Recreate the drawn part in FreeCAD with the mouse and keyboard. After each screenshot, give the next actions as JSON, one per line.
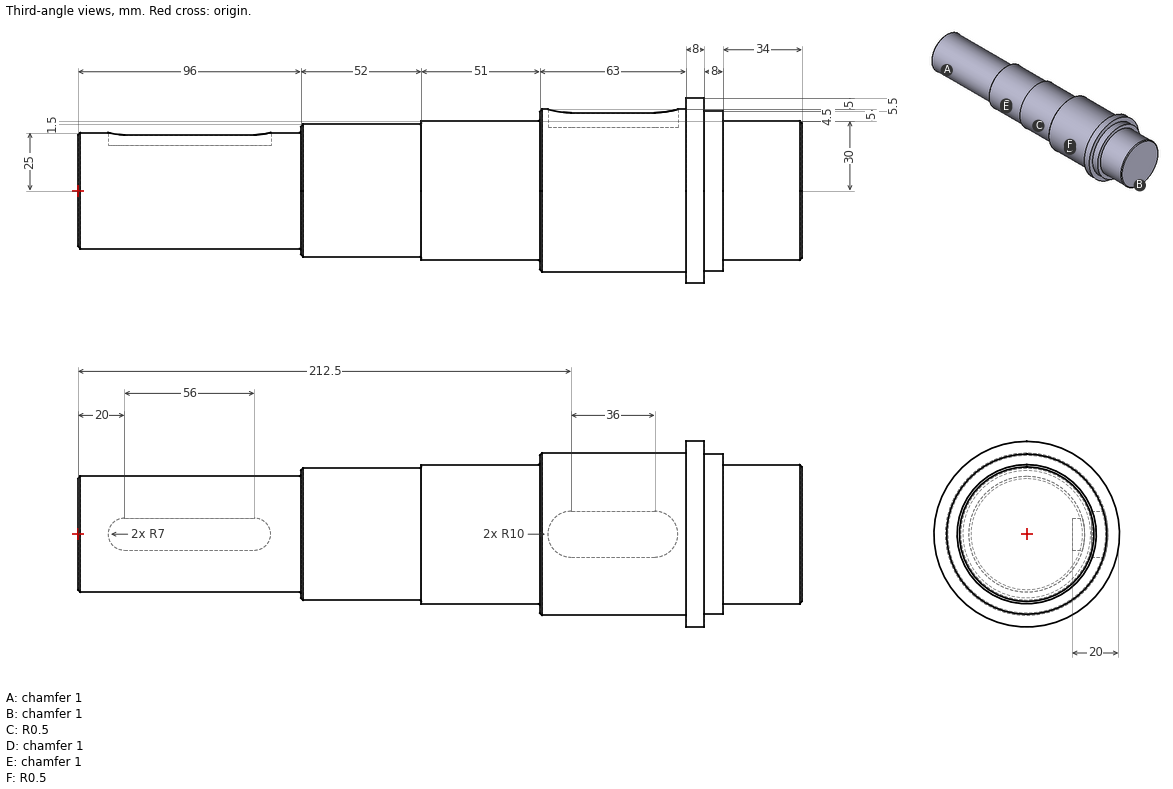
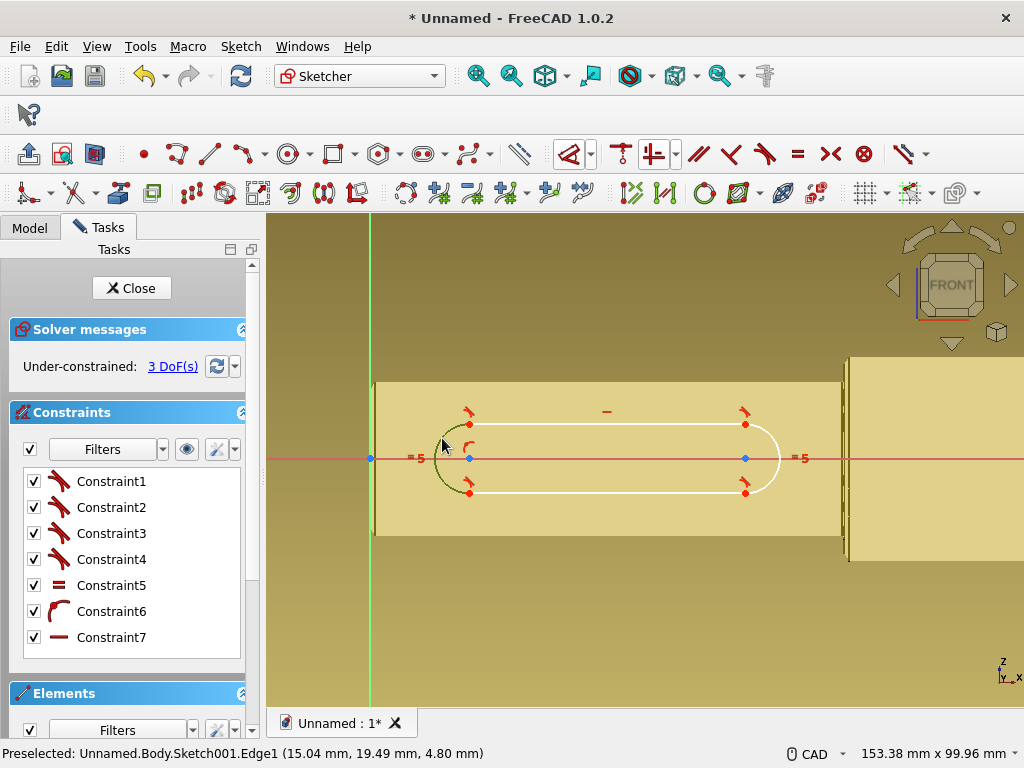
{"action": "key", "text": "k r"}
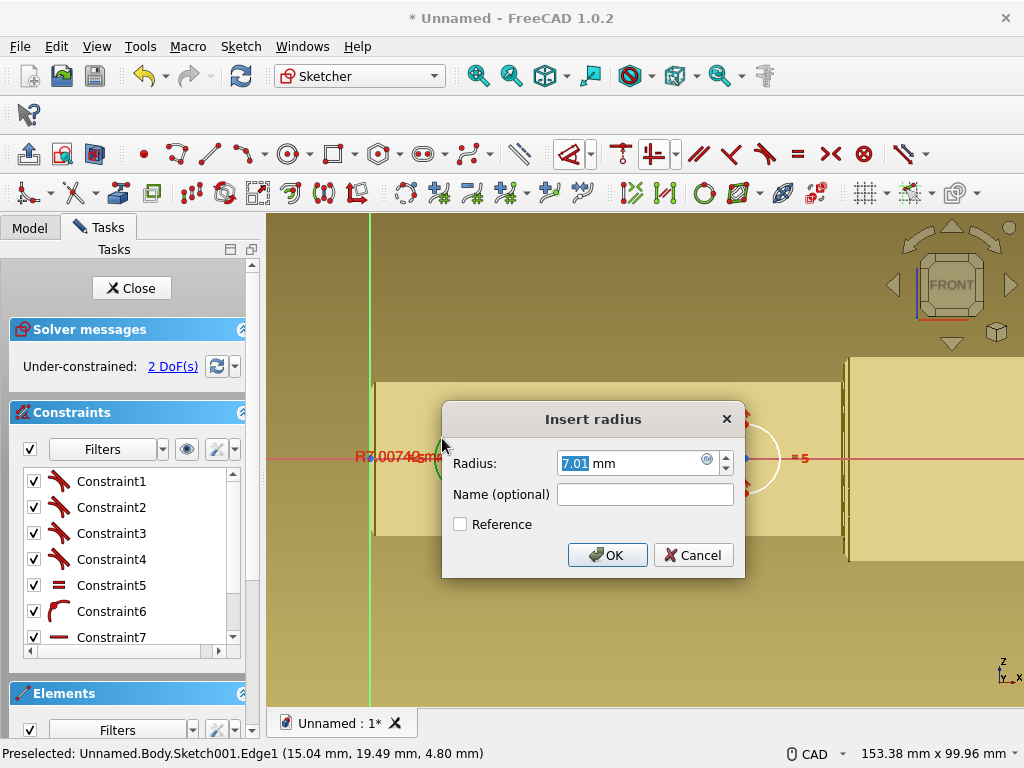
{"action": "type", "text": "7"}
{"action": "key", "text": "Return"}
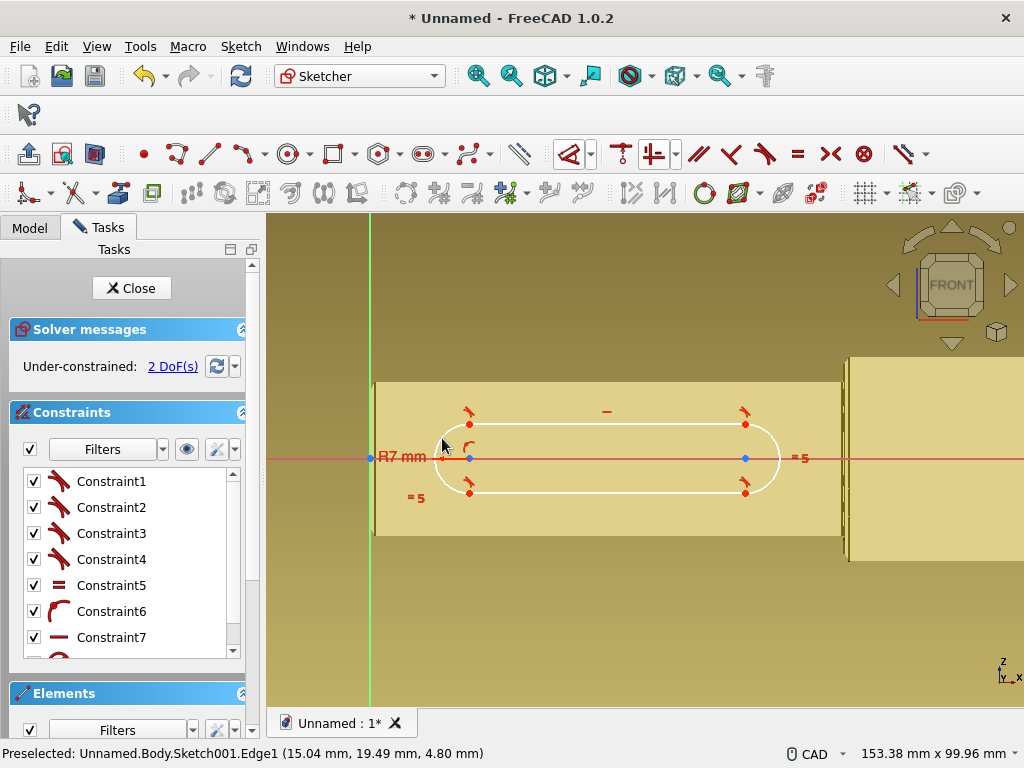
{"action": "left_click", "coordinate": [552, 424]}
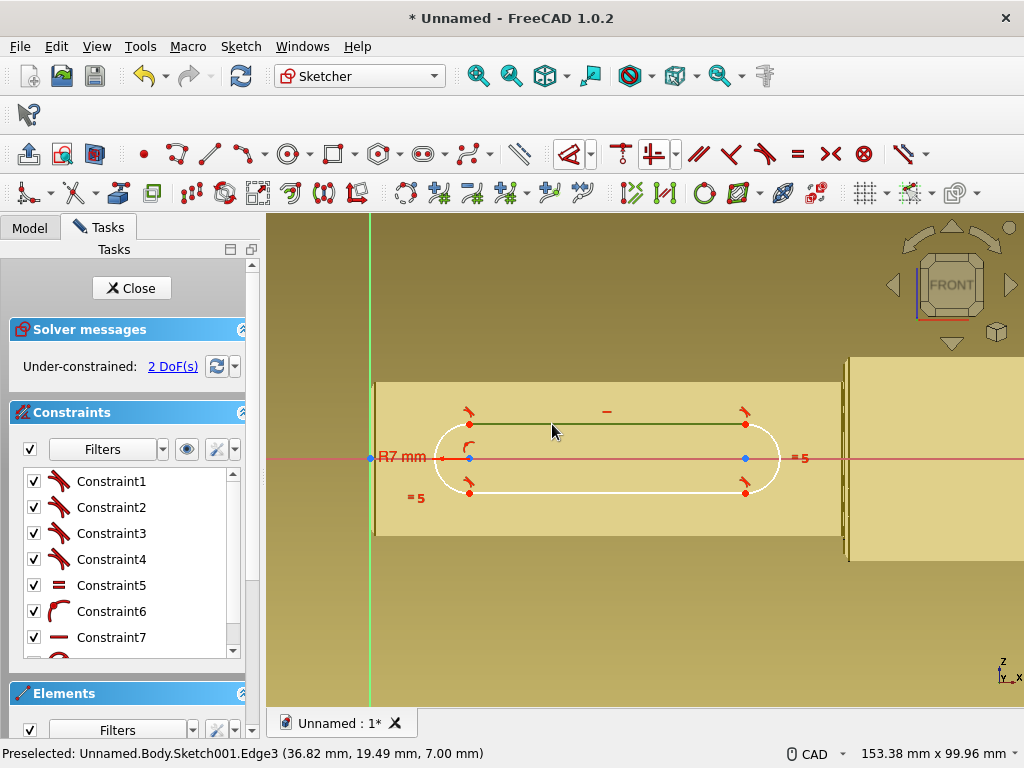
{"action": "key", "text": "l"}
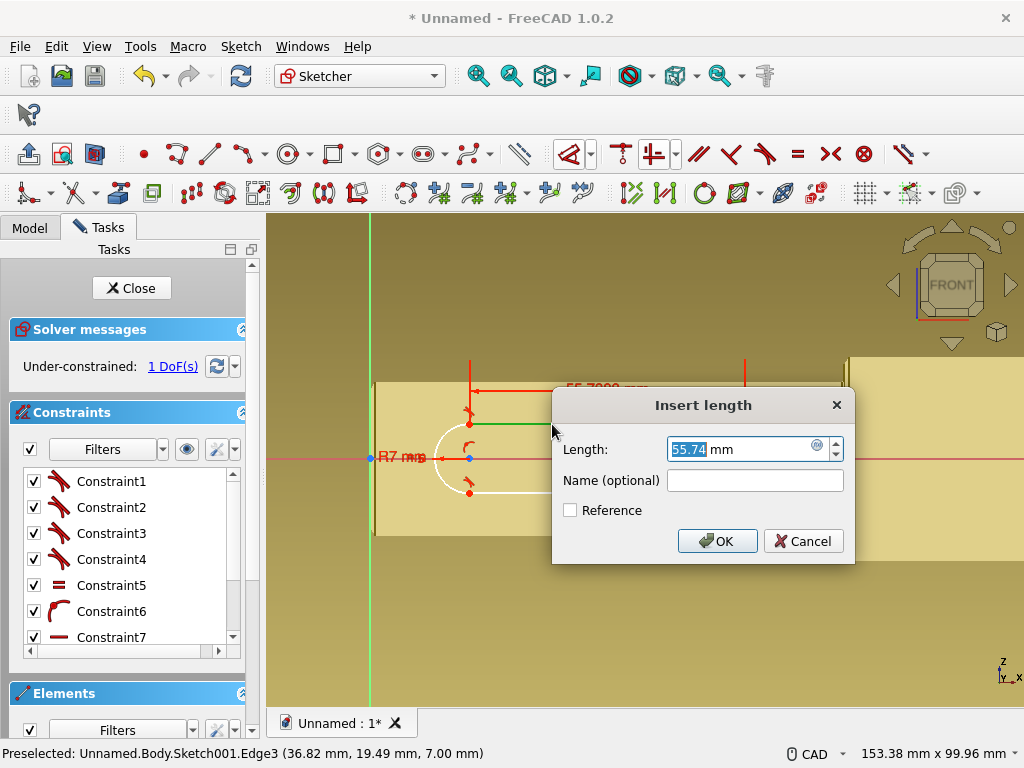
{"action": "type", "text": "56"}
{"action": "key", "text": "Return"}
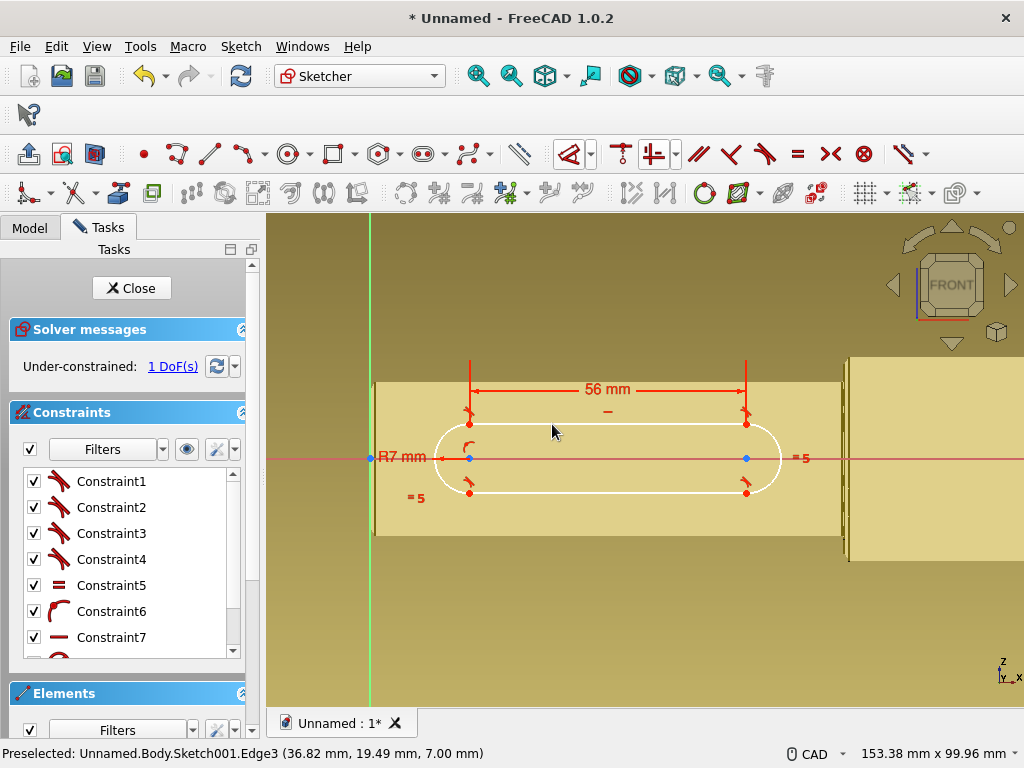
{"action": "left_click", "coordinate": [470, 424]}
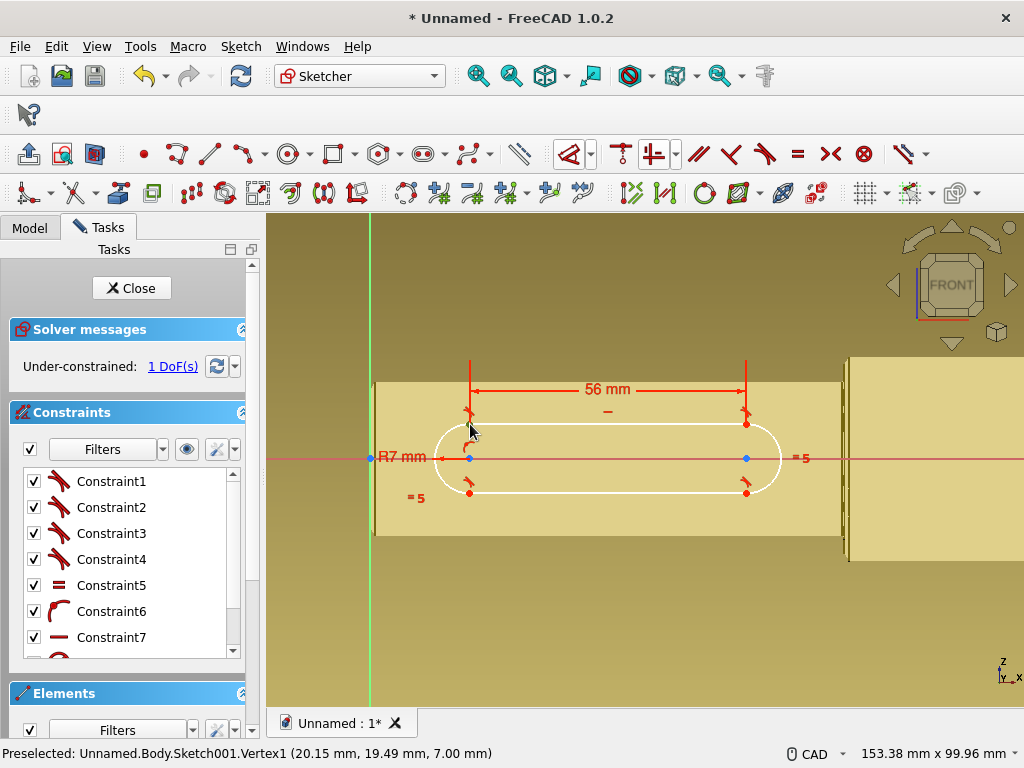
{"action": "key", "text": "l"}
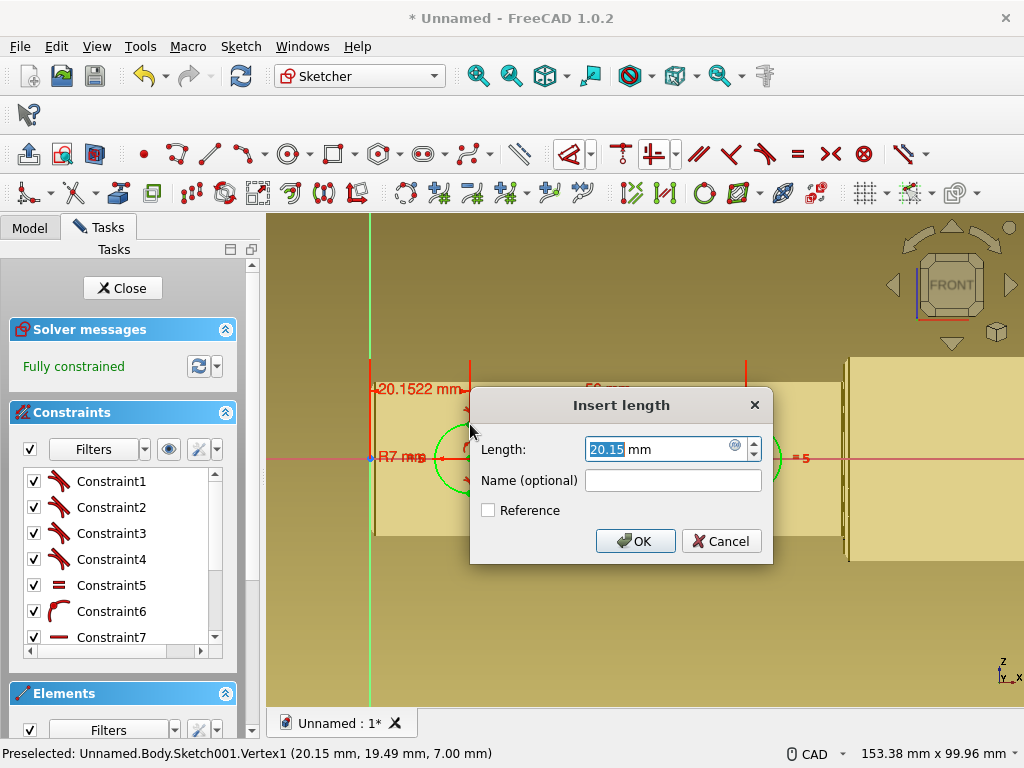
{"action": "type", "text": "20"}
{"action": "key", "text": "Return"}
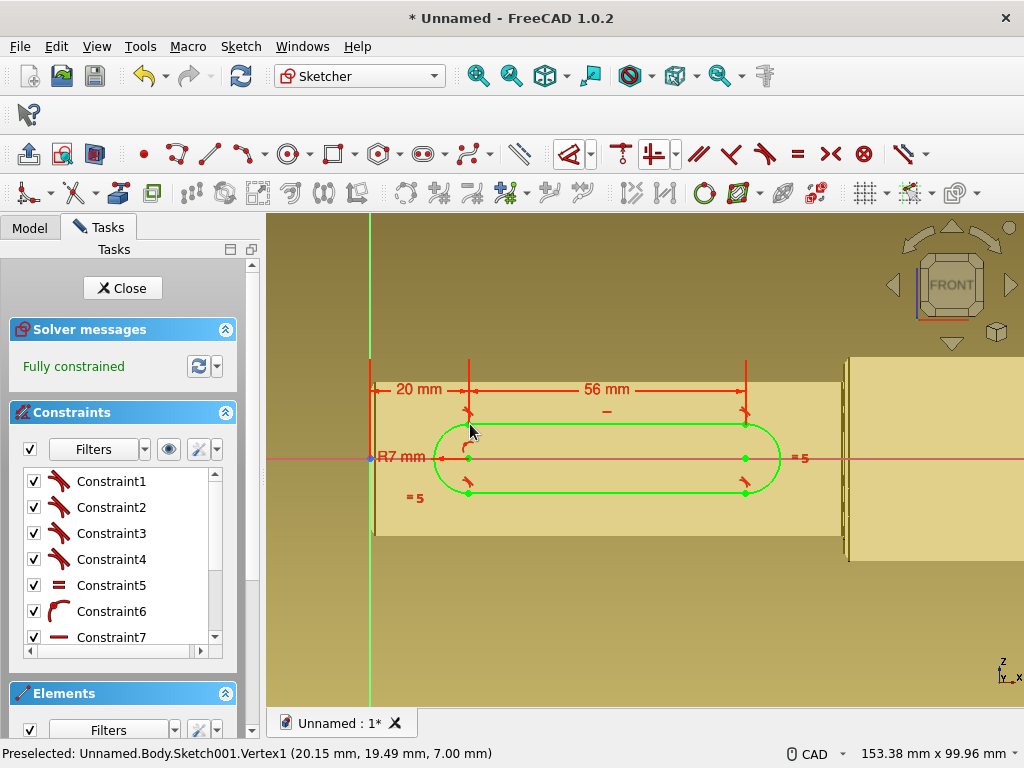
{"action": "left_click", "coordinate": [123, 288]}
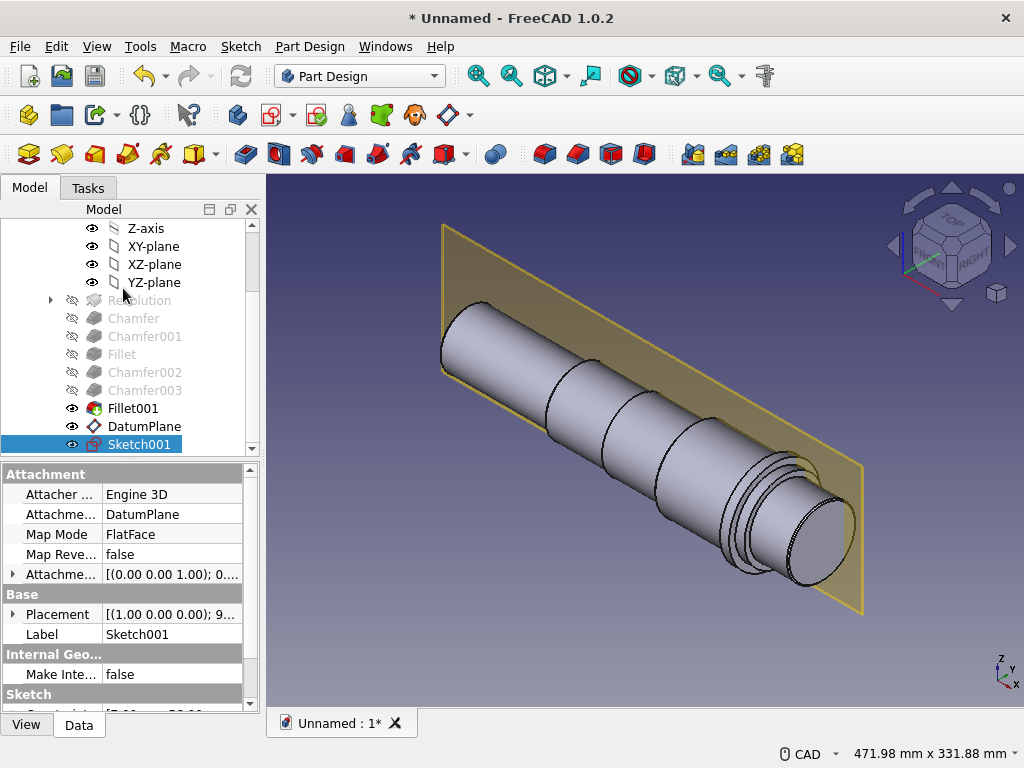
{"action": "left_click", "coordinate": [246, 154]}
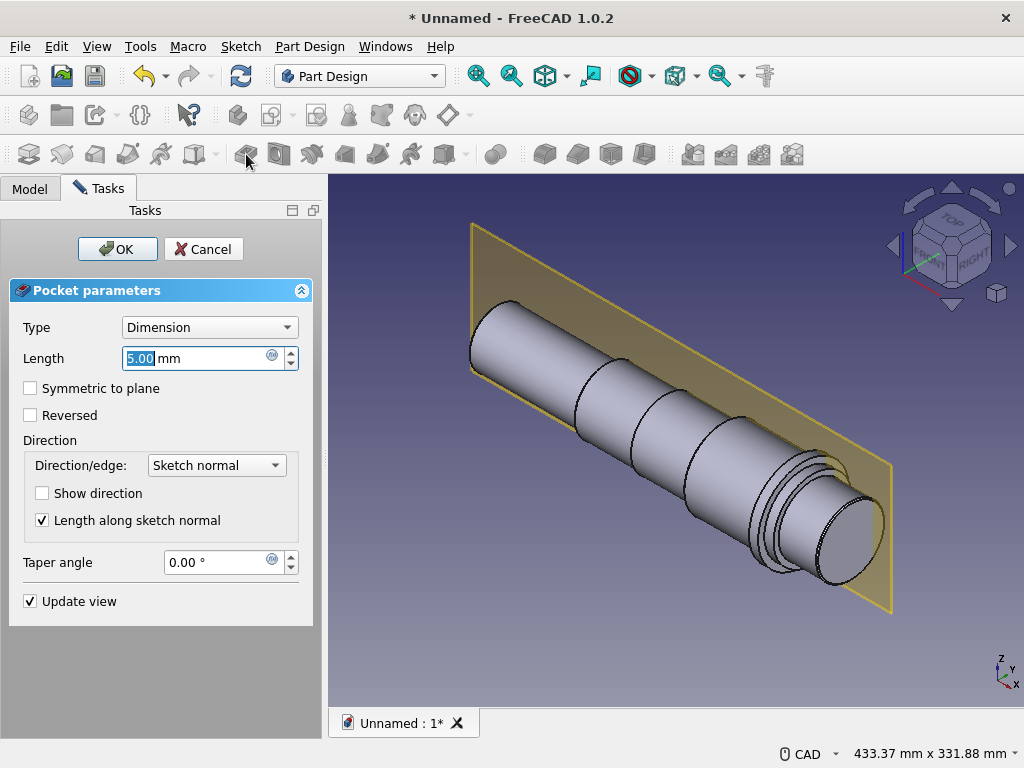
{"action": "type", "text": "20"}
{"action": "key", "text": "Tab"}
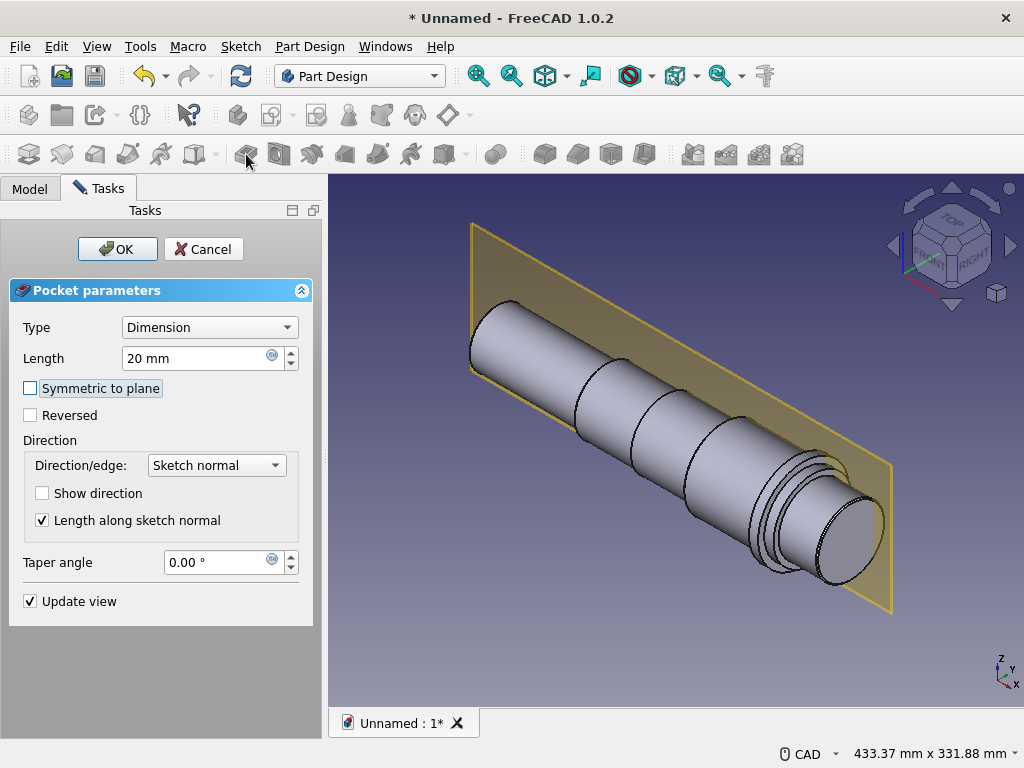
{"action": "left_click", "coordinate": [118, 249]}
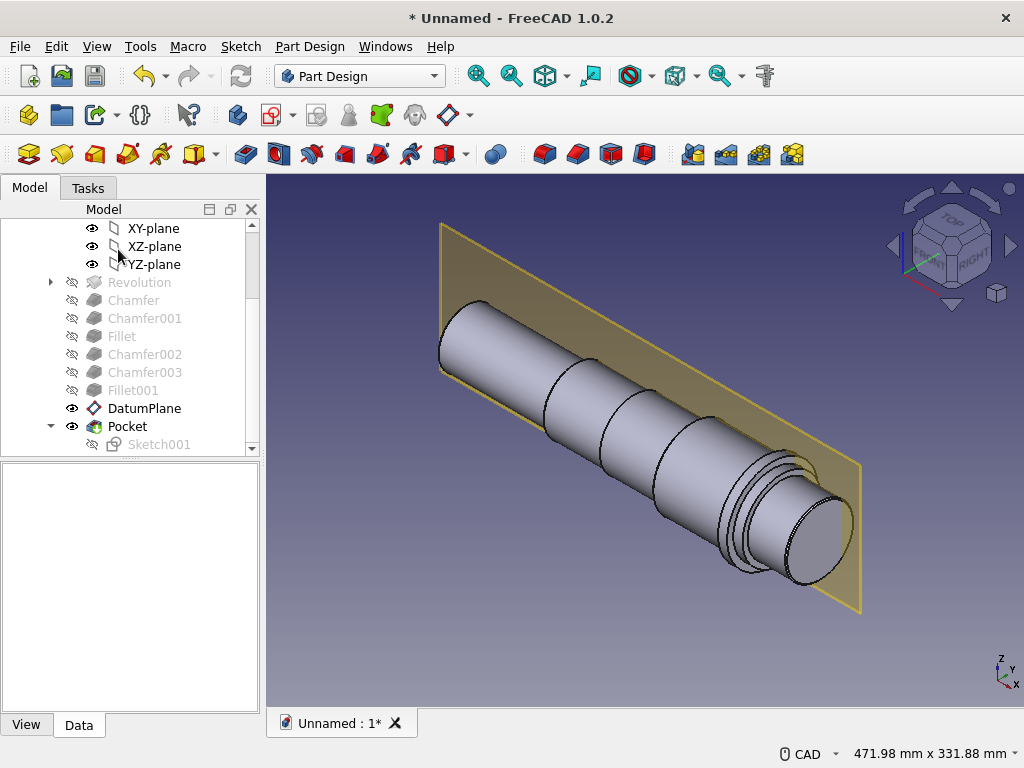
{"action": "left_click", "coordinate": [117, 408]}
{"action": "key", "text": "space"}